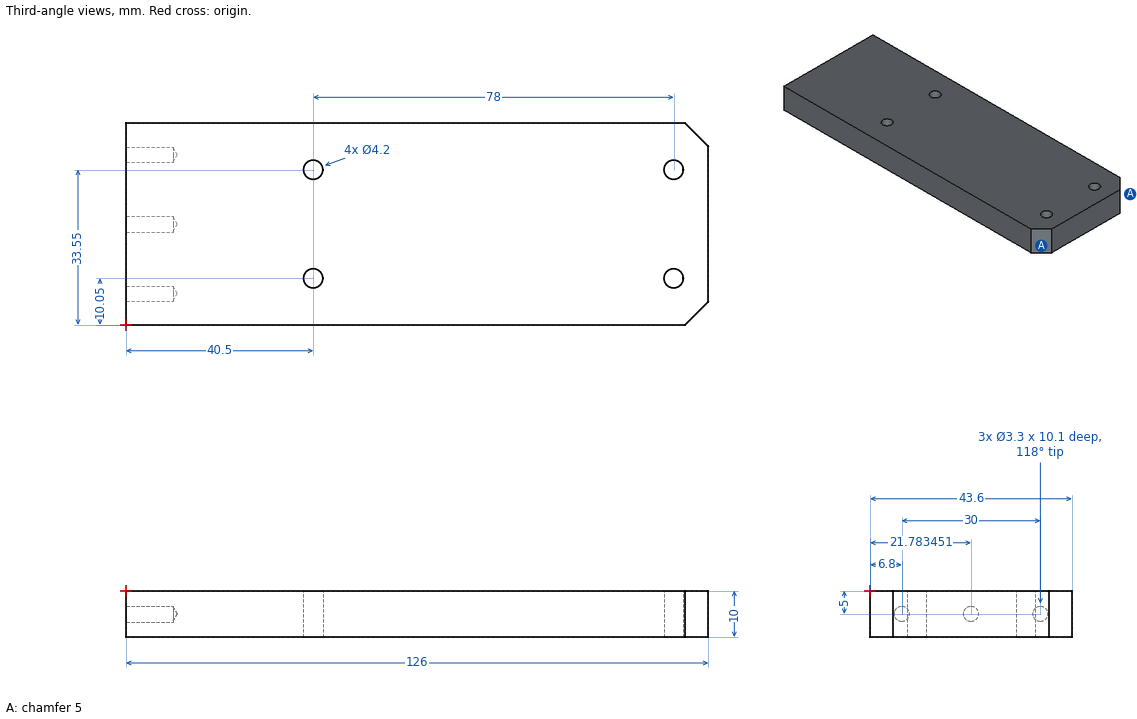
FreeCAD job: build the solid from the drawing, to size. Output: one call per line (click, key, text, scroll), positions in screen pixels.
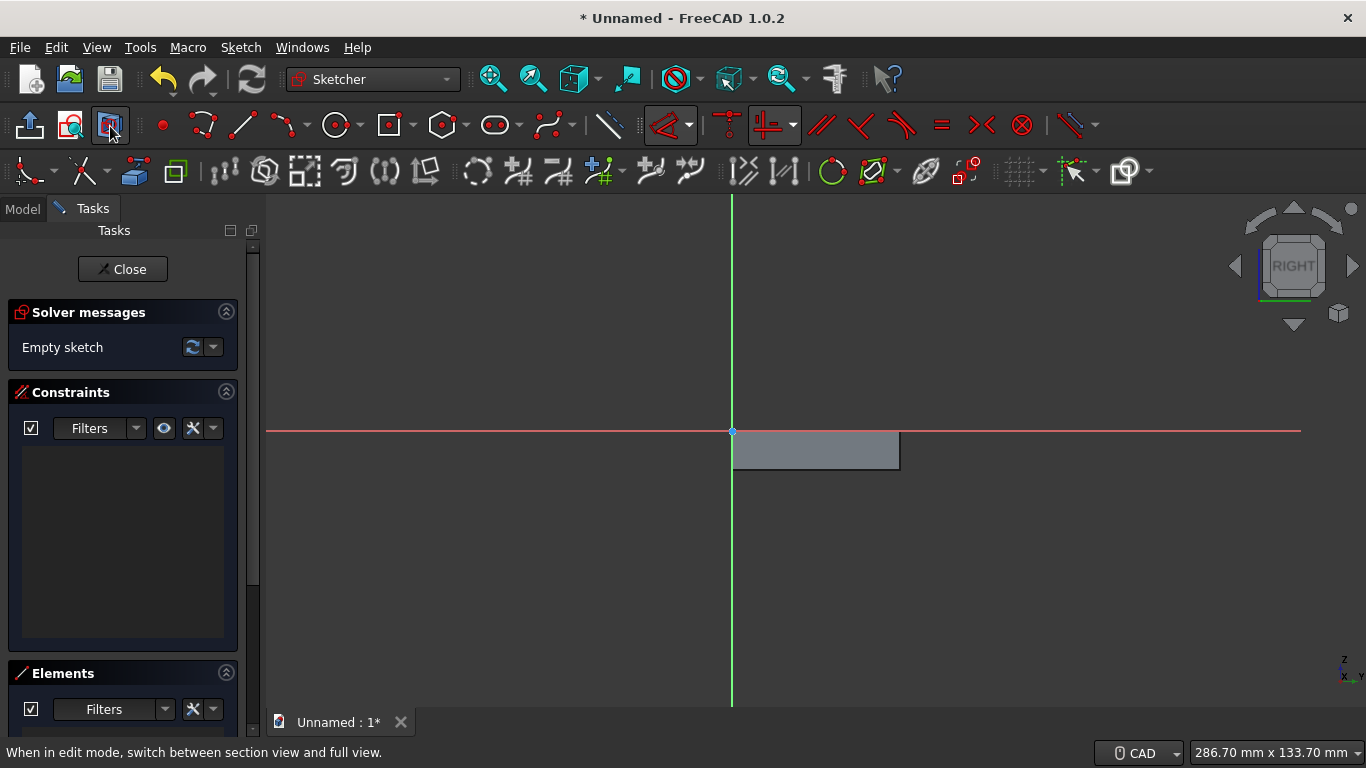
scroll(825, 442, up, 7)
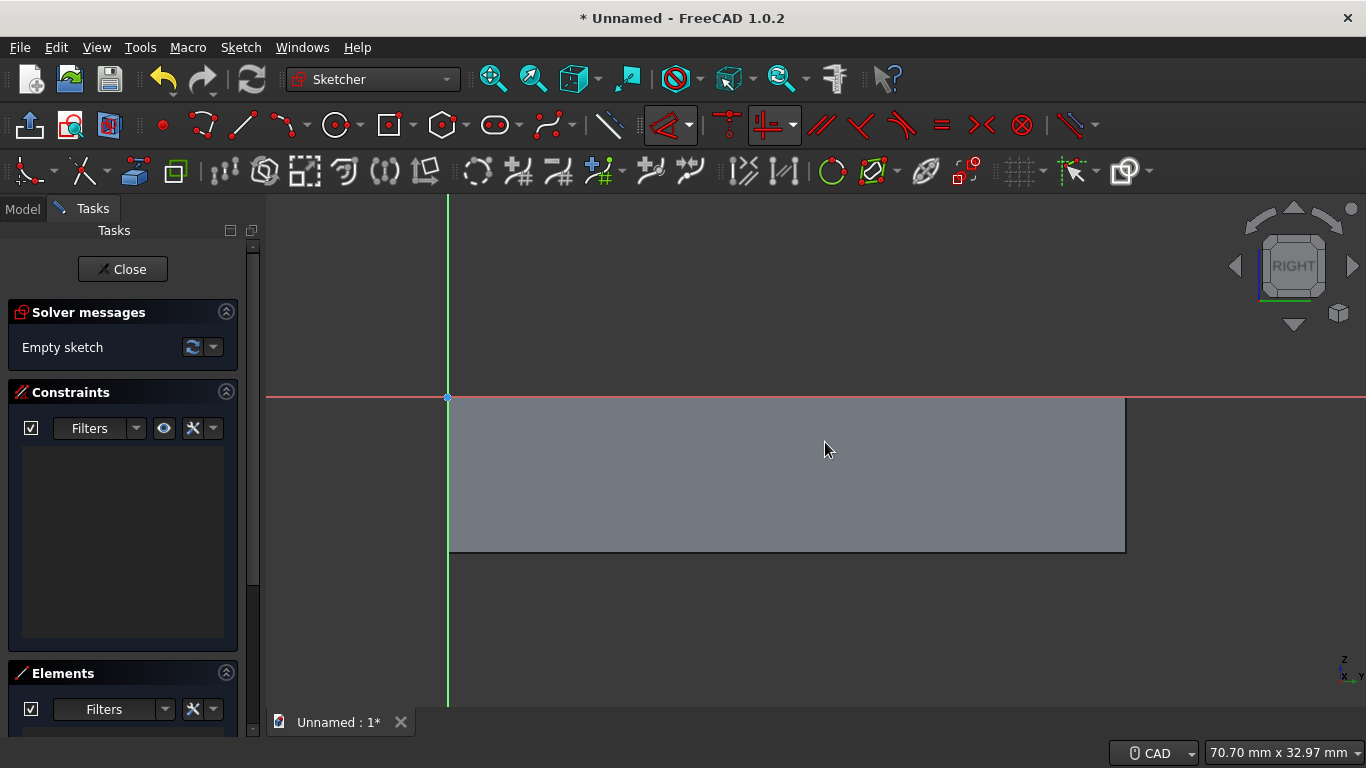
click(336, 126)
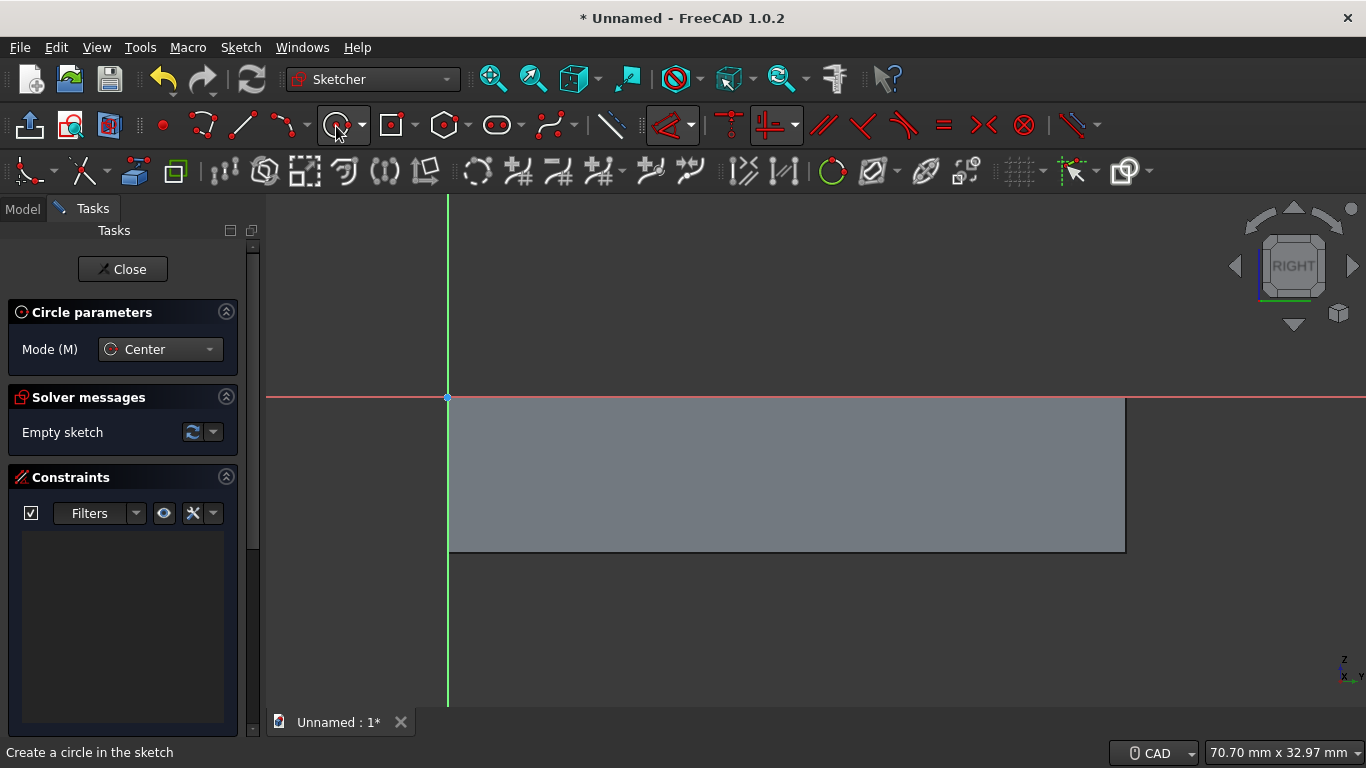
click(1020, 475)
move(1038, 457)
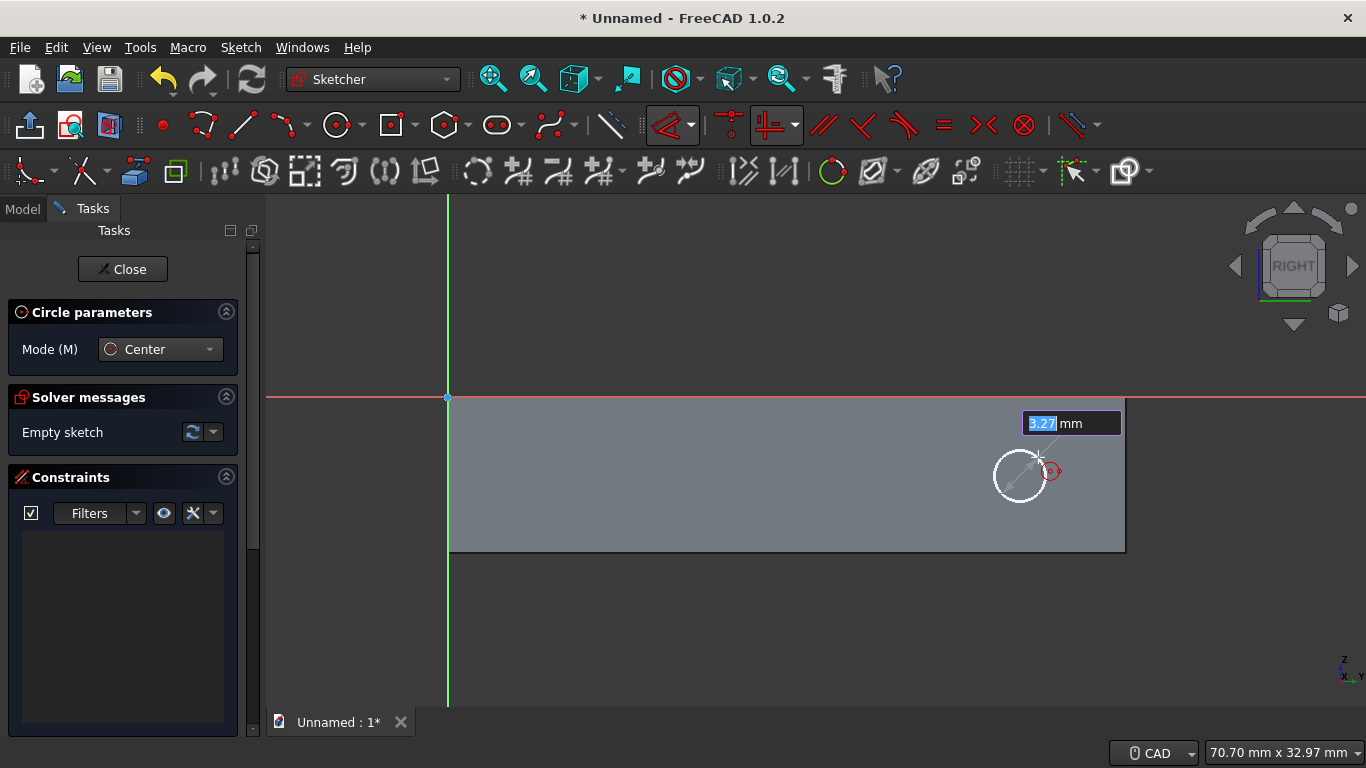
text(3.3)
key(Return)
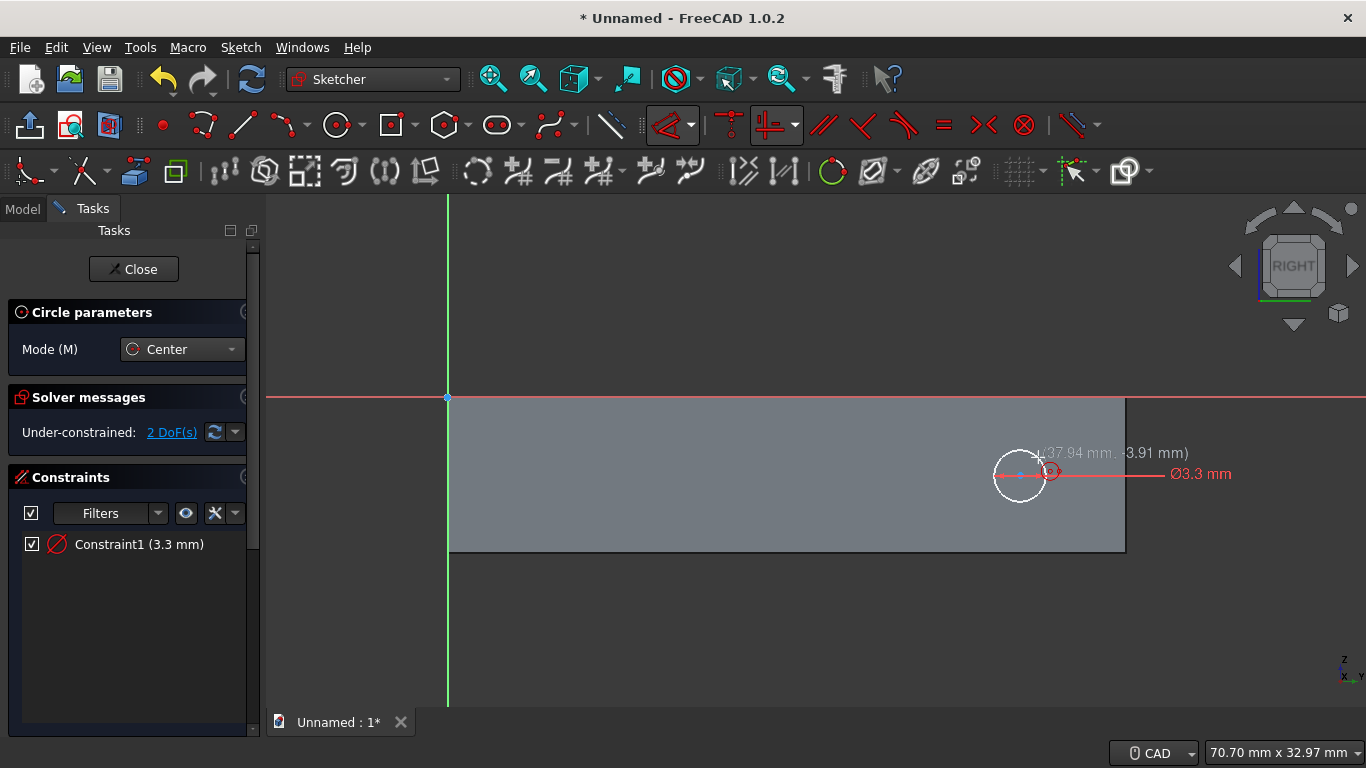
click(787, 475)
move(805, 457)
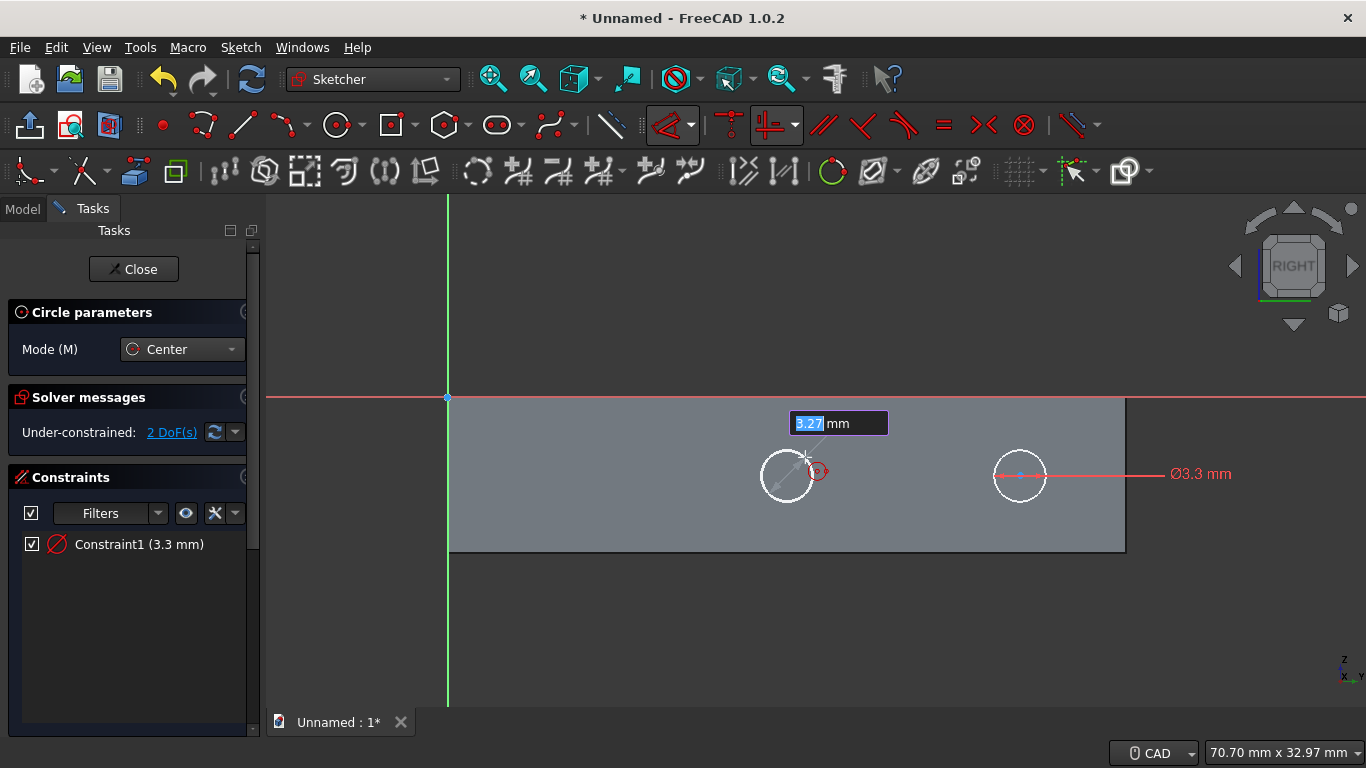
text(3.3)
key(Return)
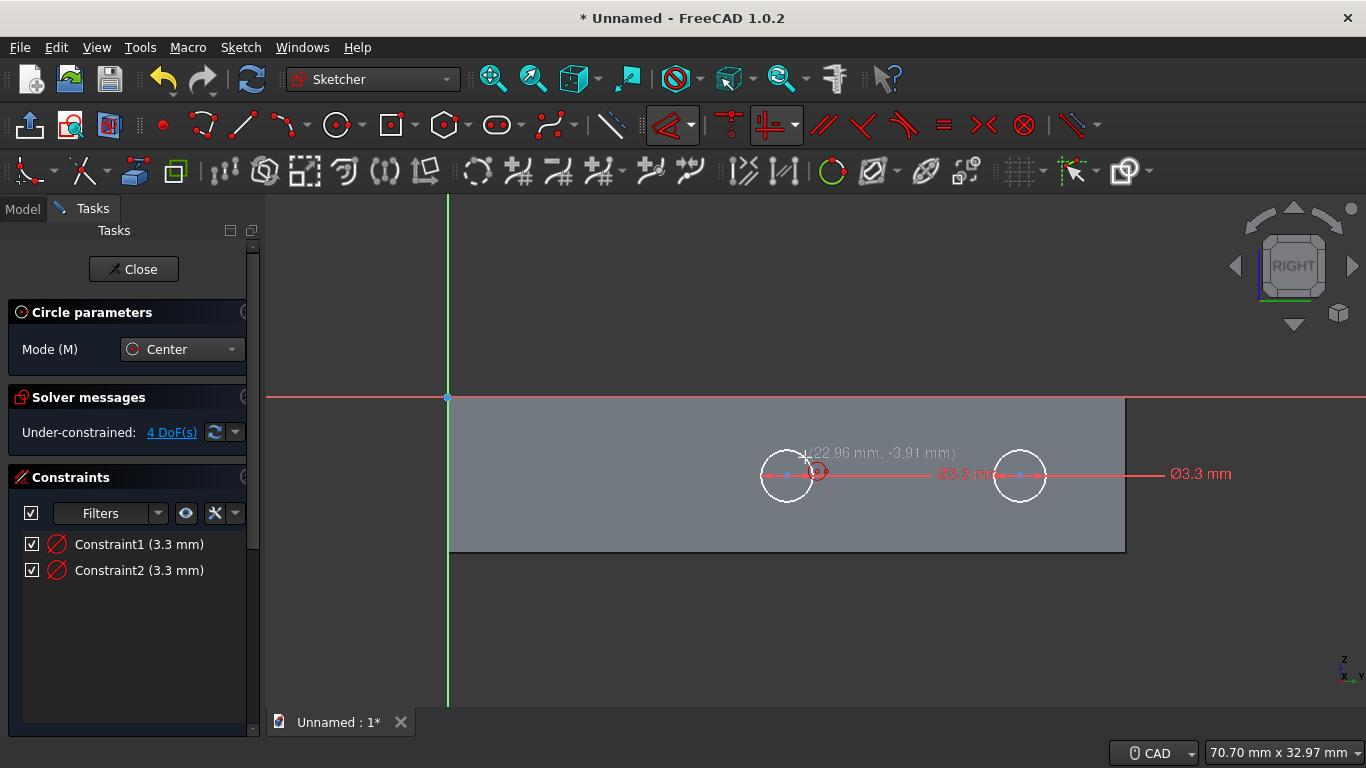
click(554, 475)
move(572, 457)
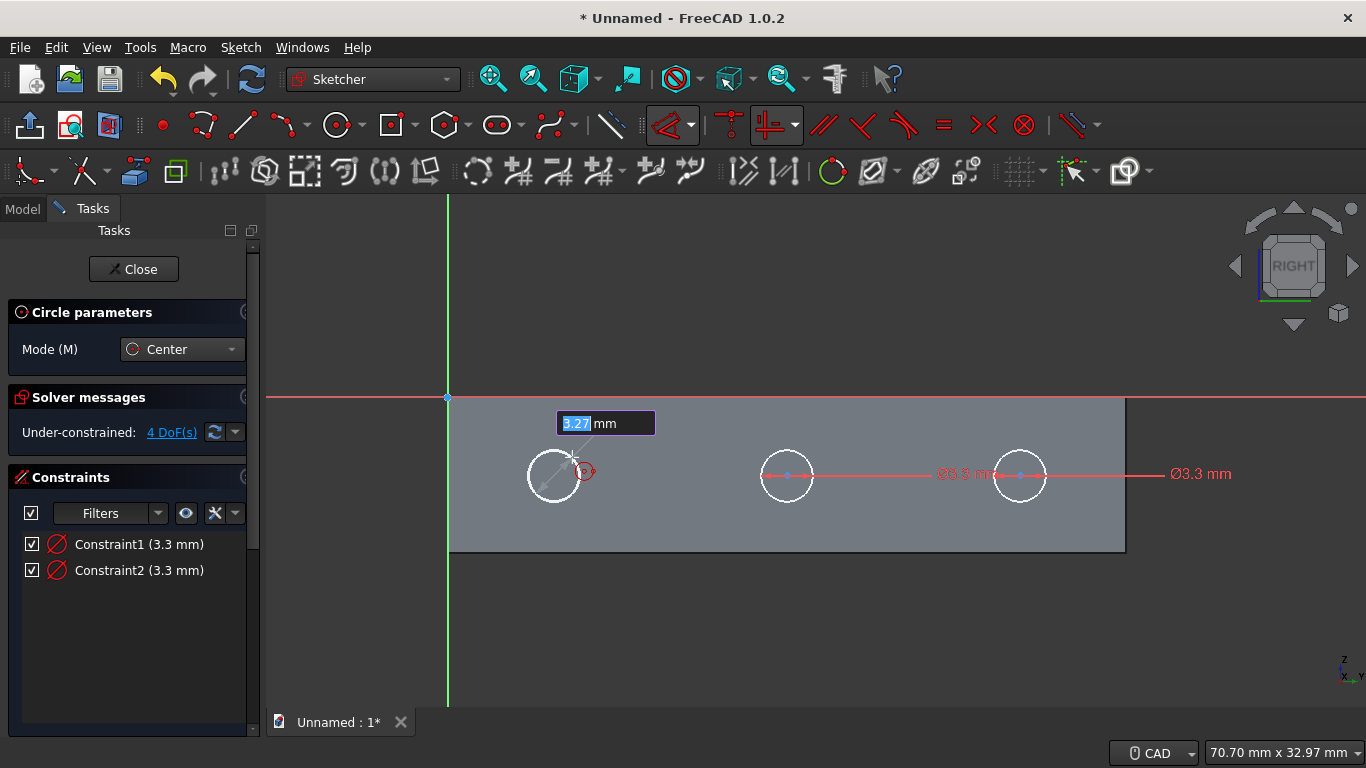
text(3.3)
key(Return)
key(Escape)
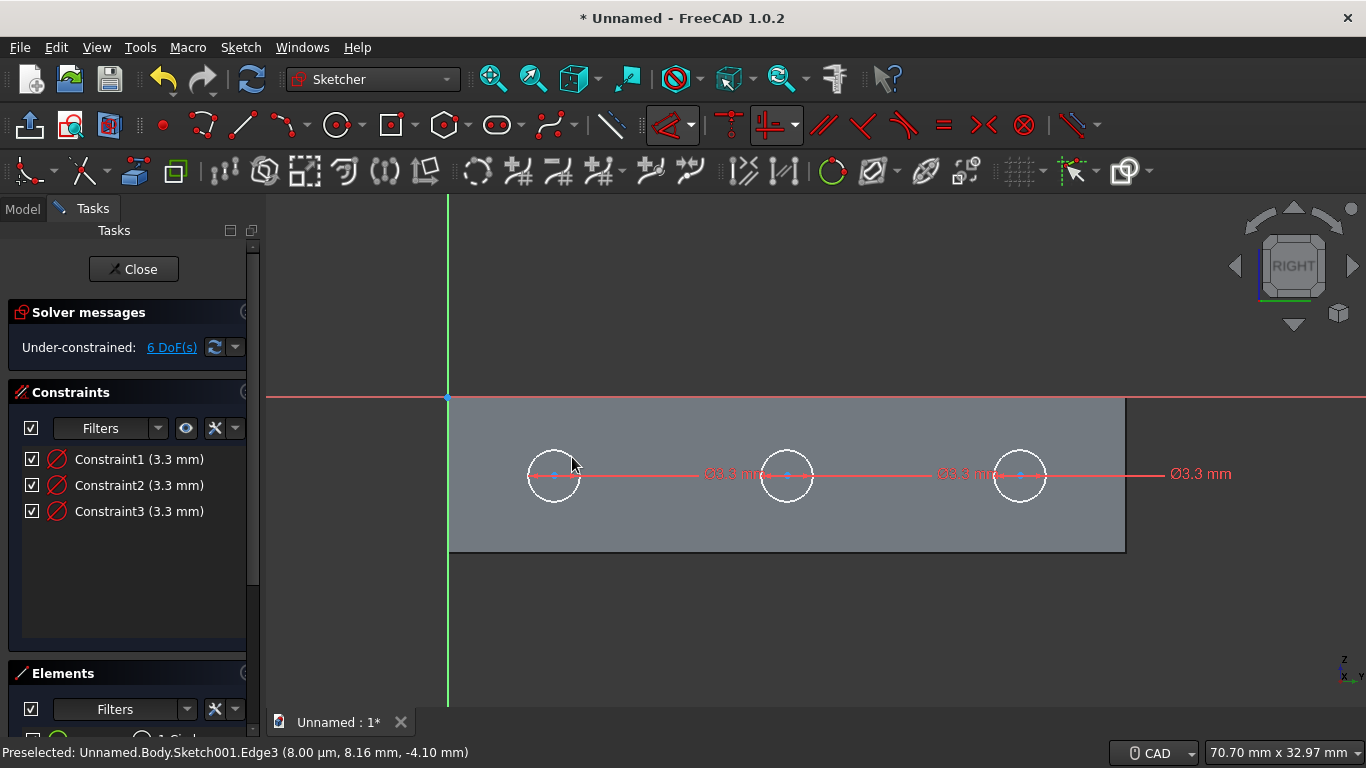
click(1020, 476)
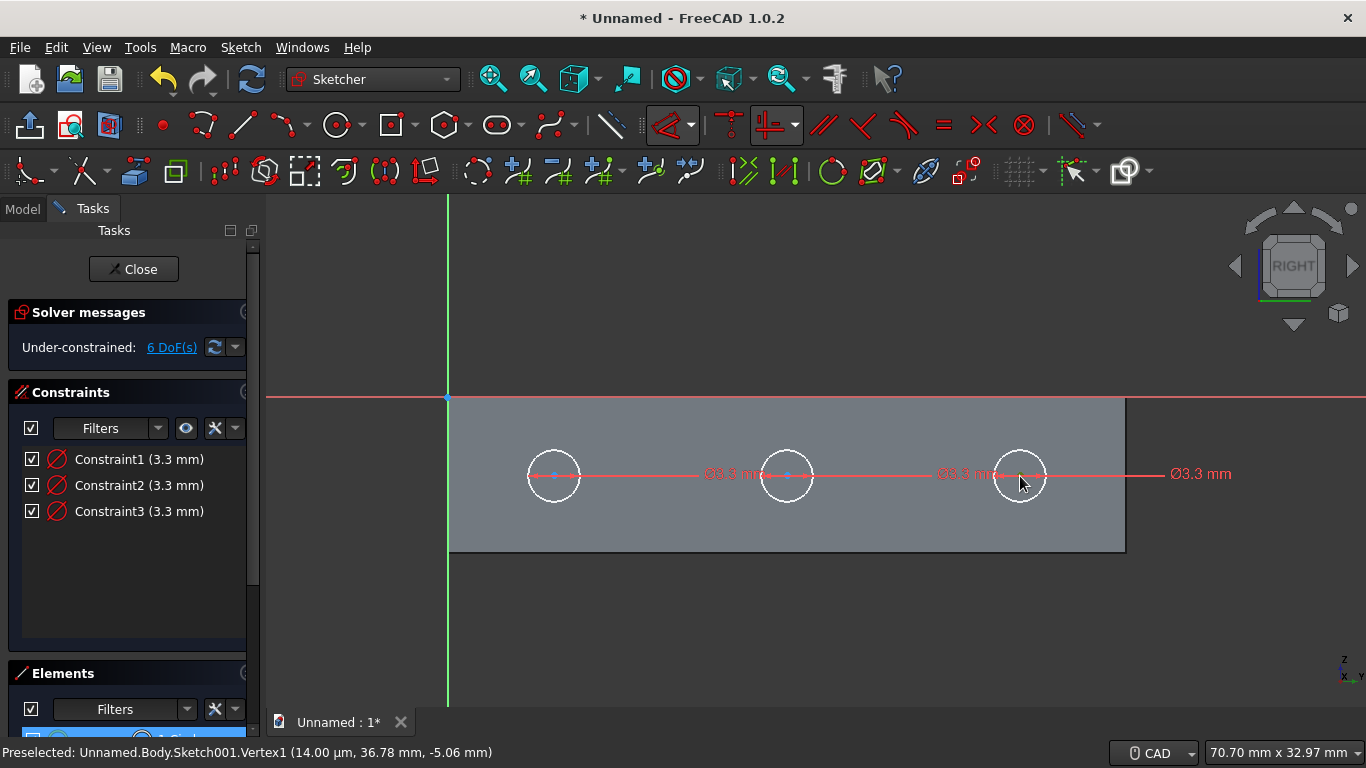
click(787, 476)